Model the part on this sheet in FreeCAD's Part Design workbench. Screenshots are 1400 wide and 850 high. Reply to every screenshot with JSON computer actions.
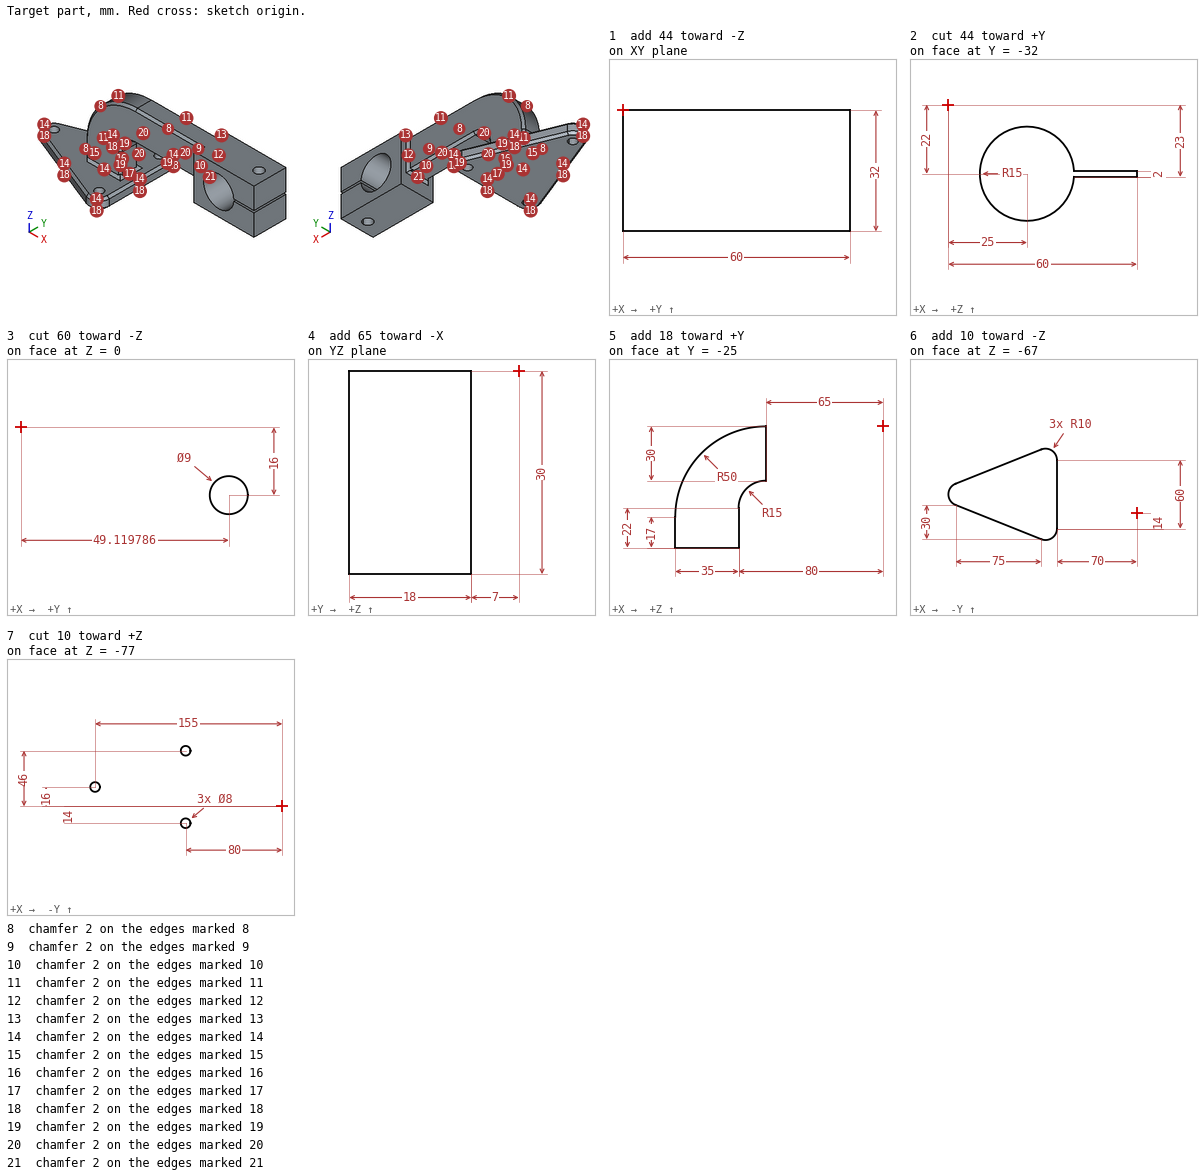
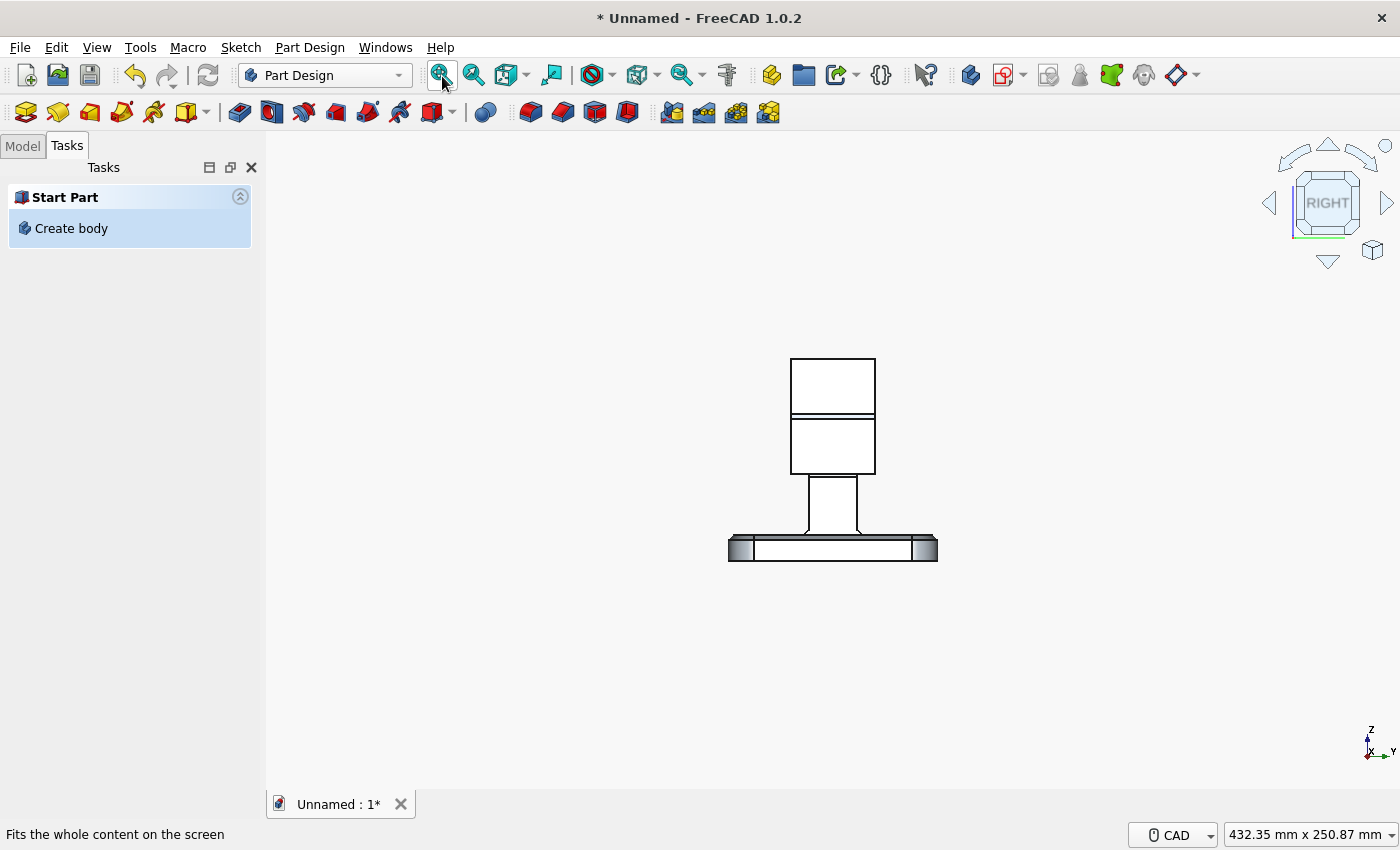
{"action": "key", "text": "5"}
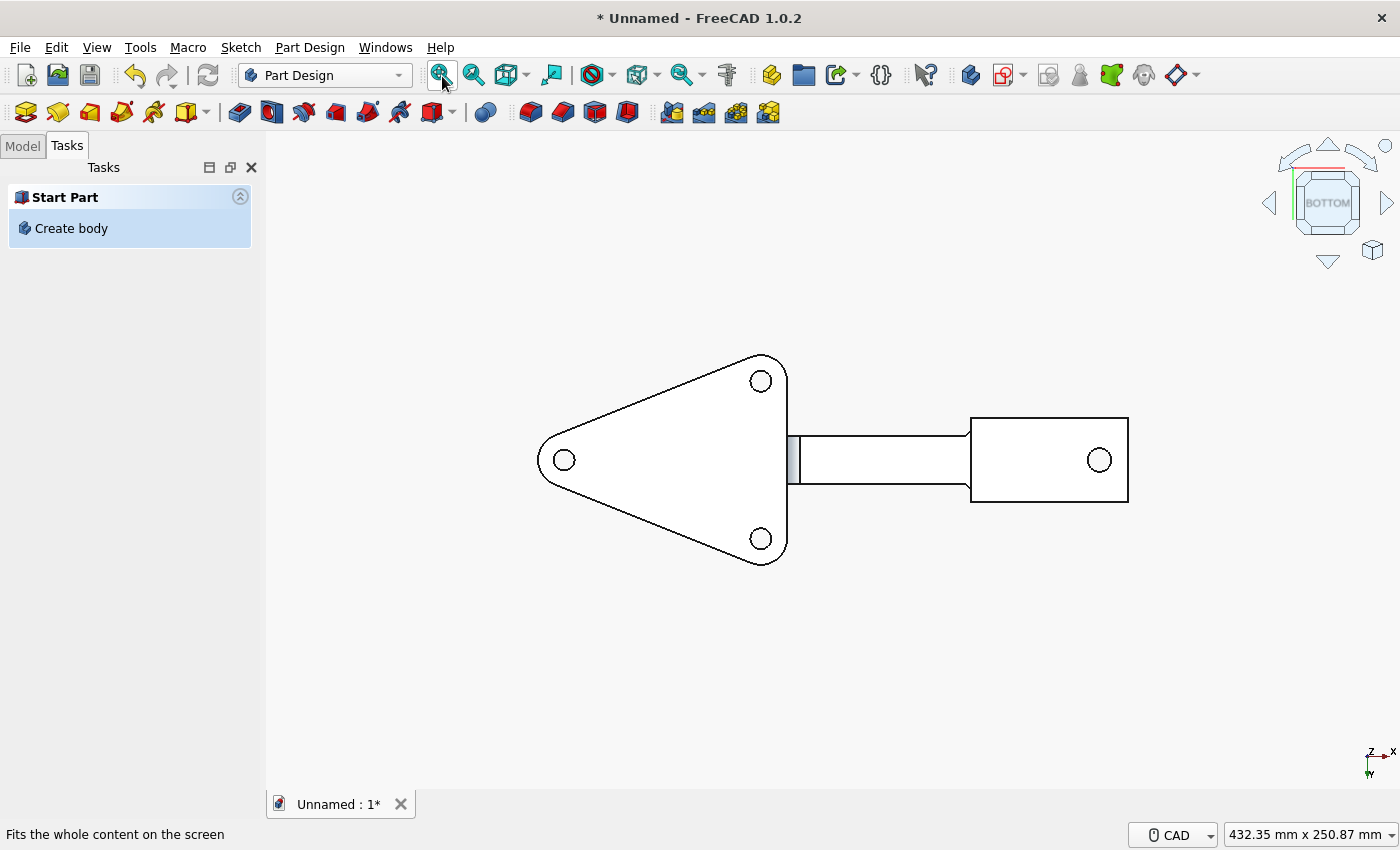
{"action": "key", "text": "4"}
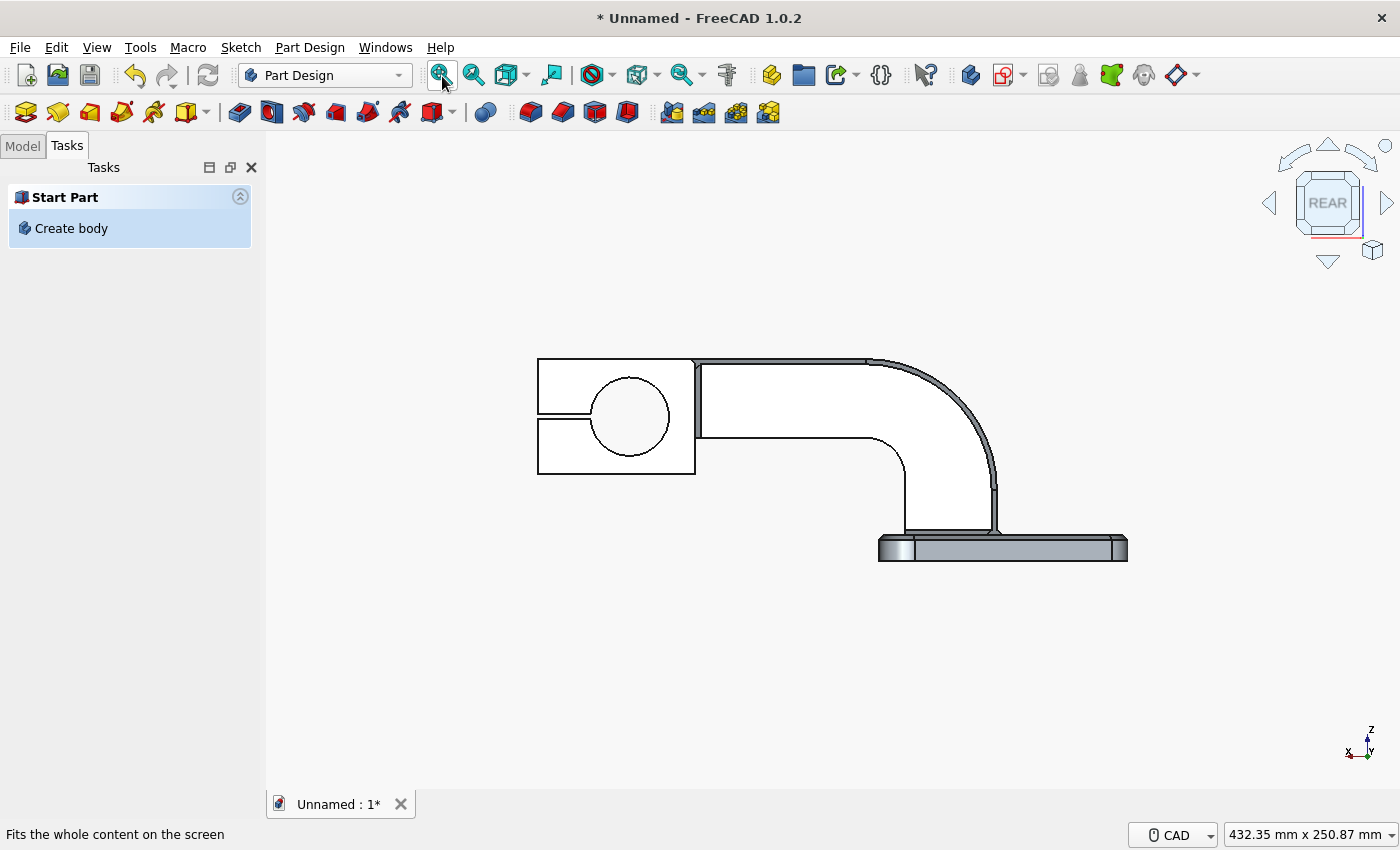
{"action": "key", "text": "6"}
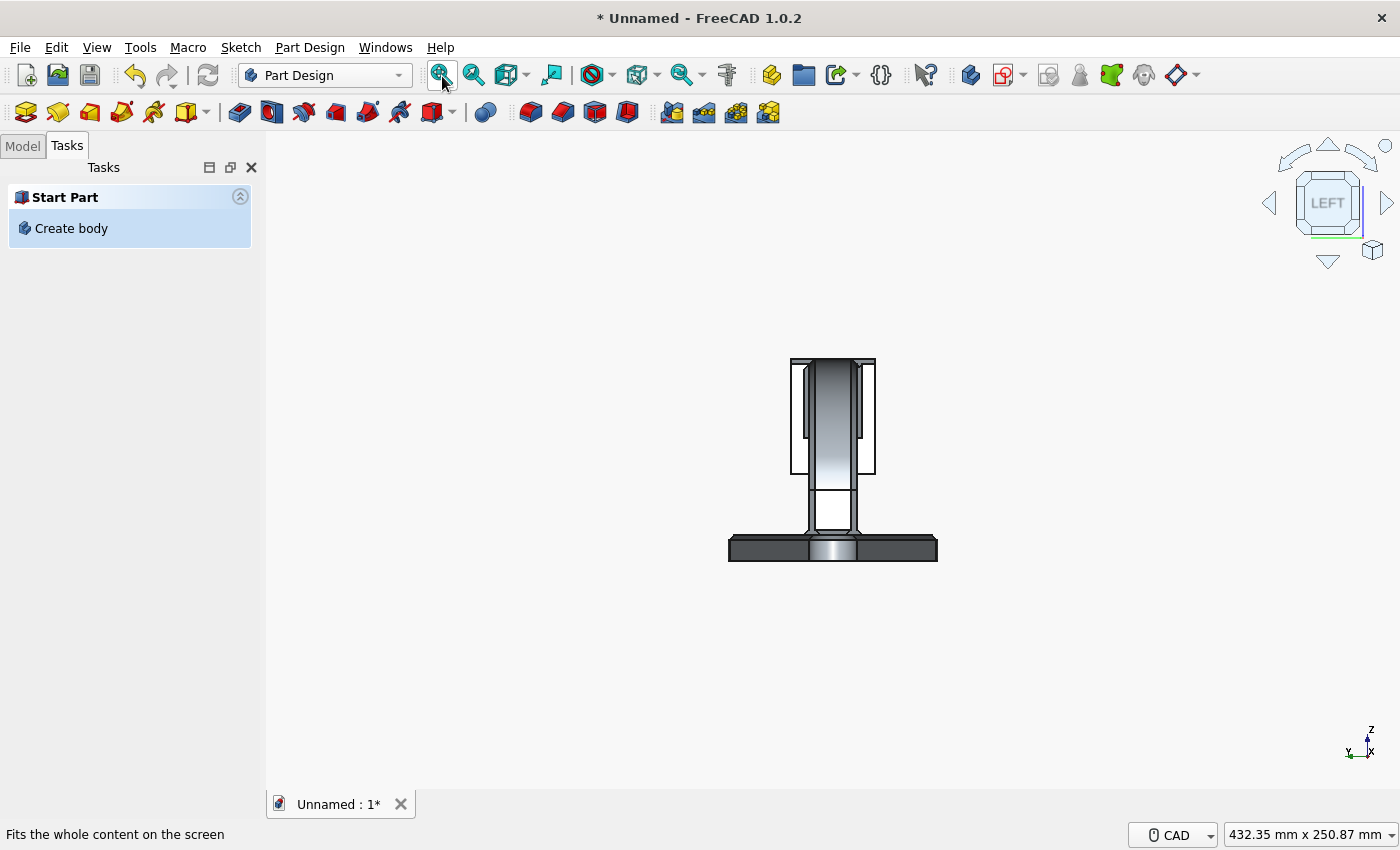
{"action": "left_click", "coordinate": [442, 76]}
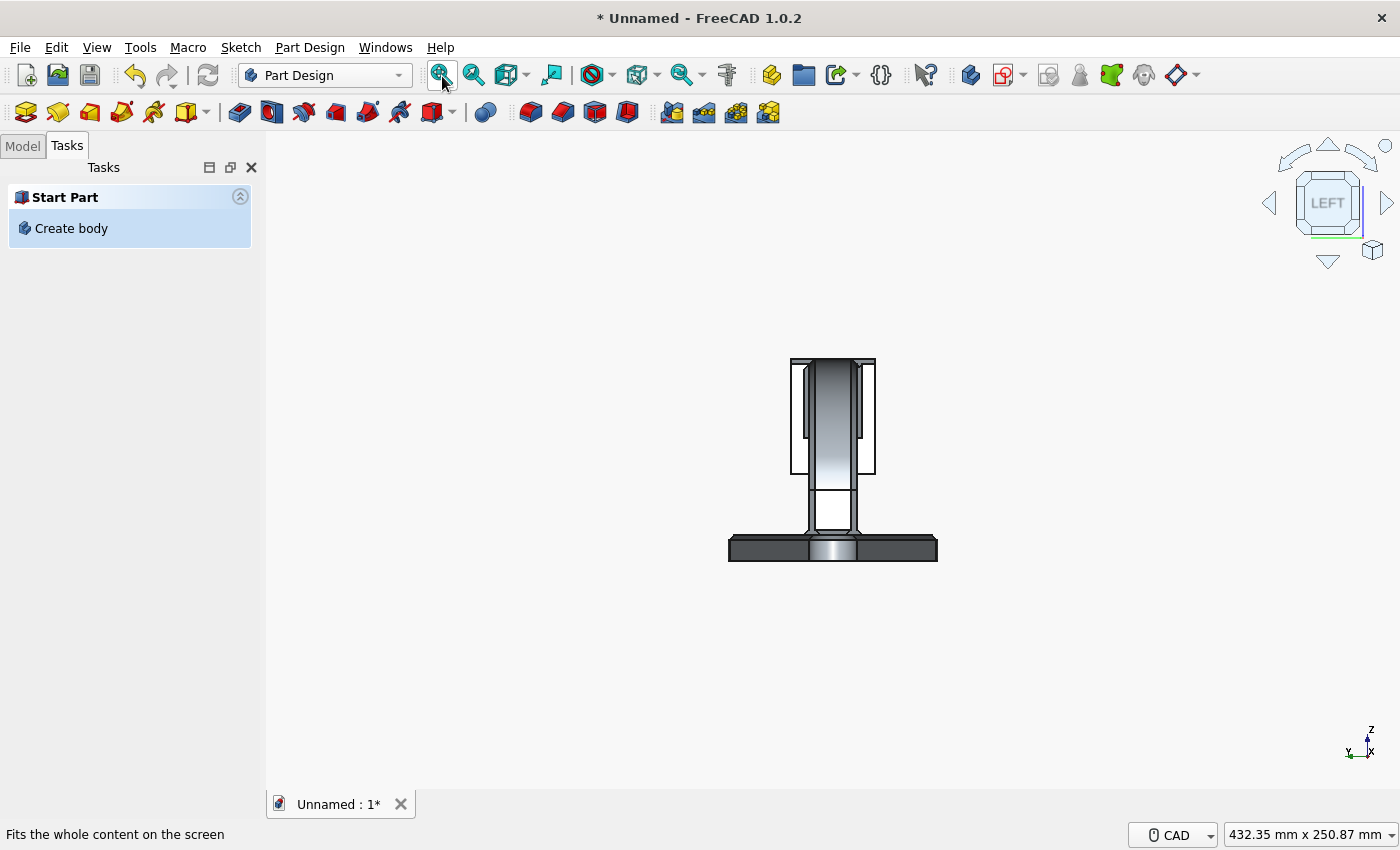
{"action": "key", "text": "v 3"}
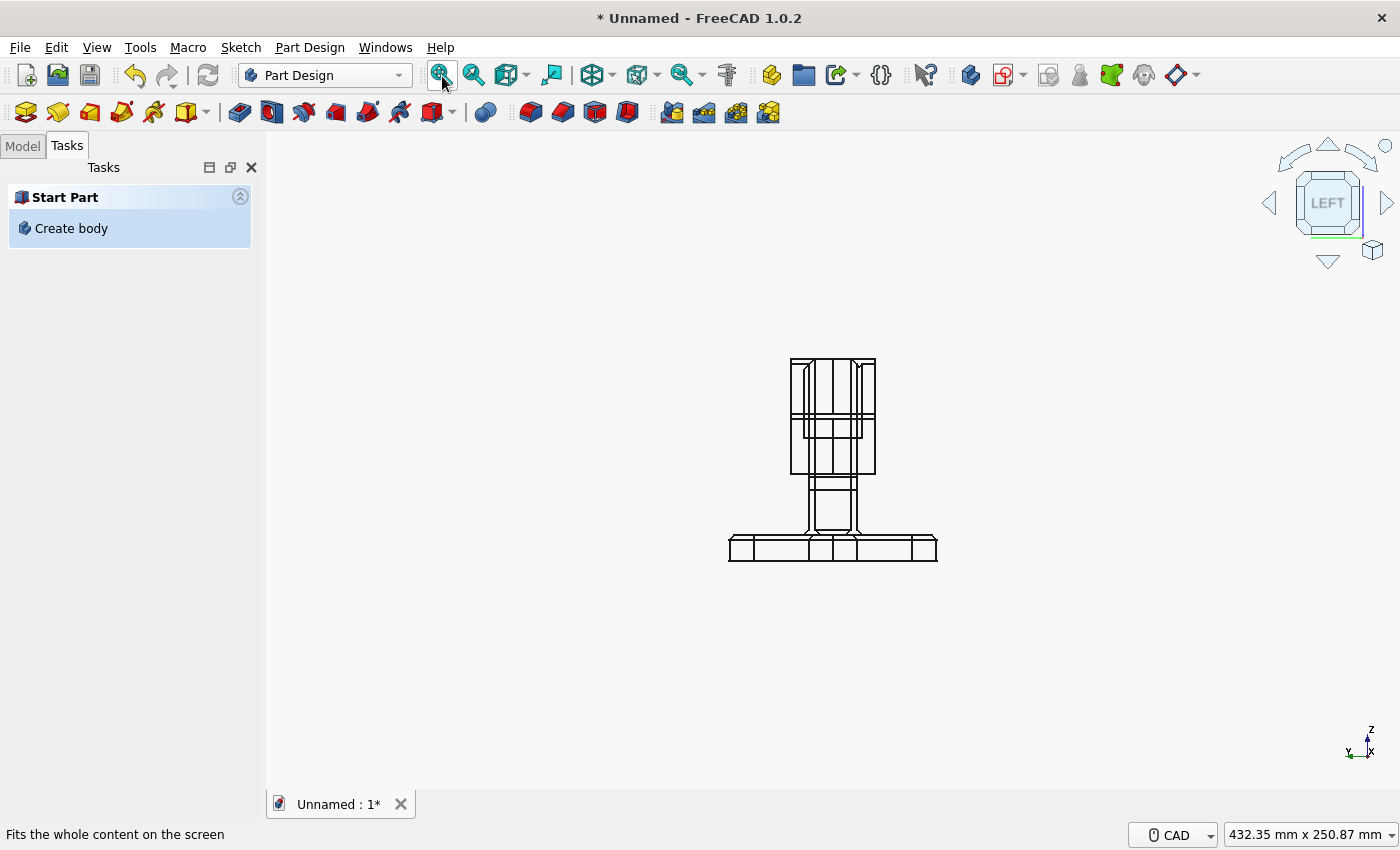
{"action": "key", "text": "0"}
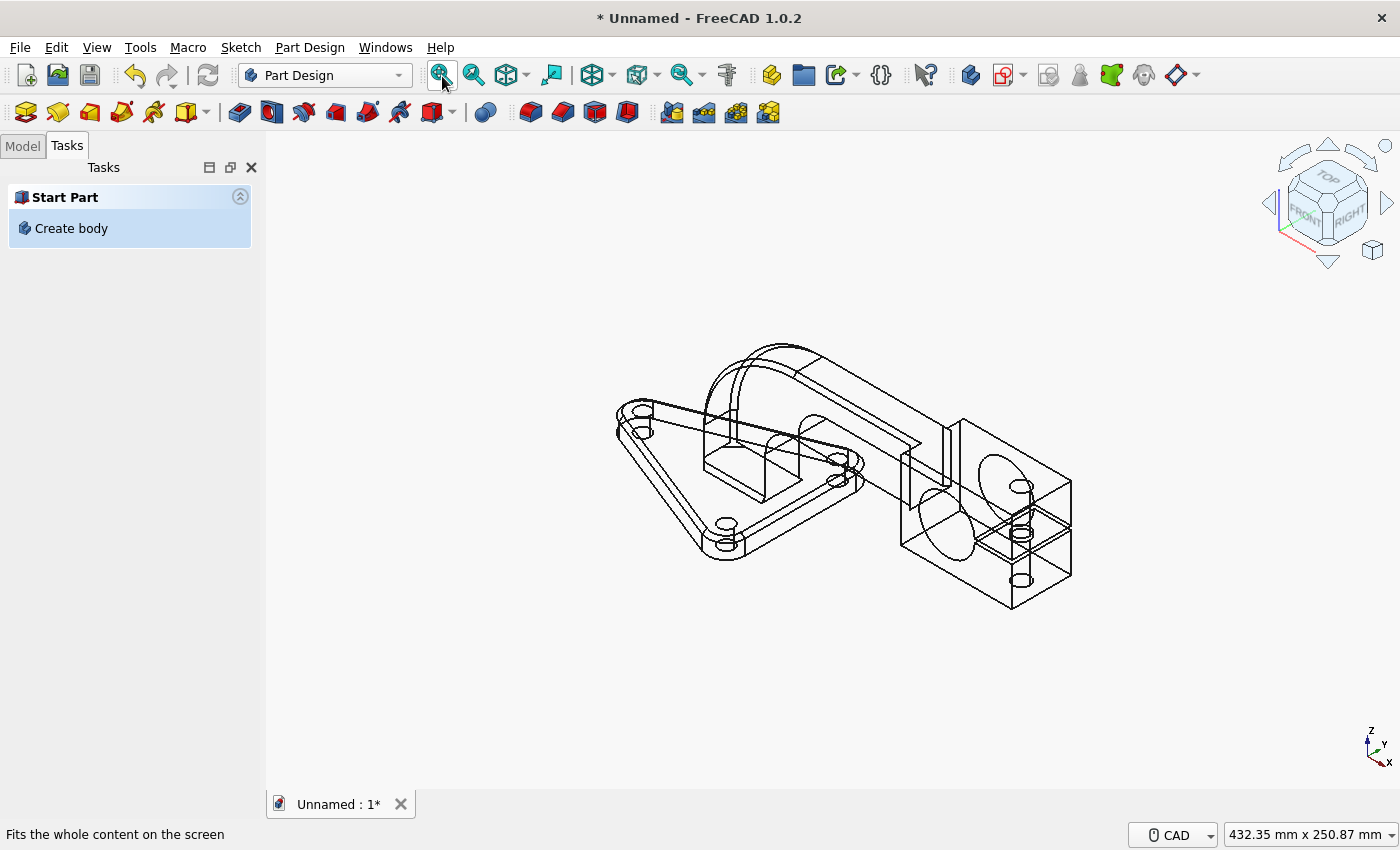
{"action": "left_click", "coordinate": [782, 491]}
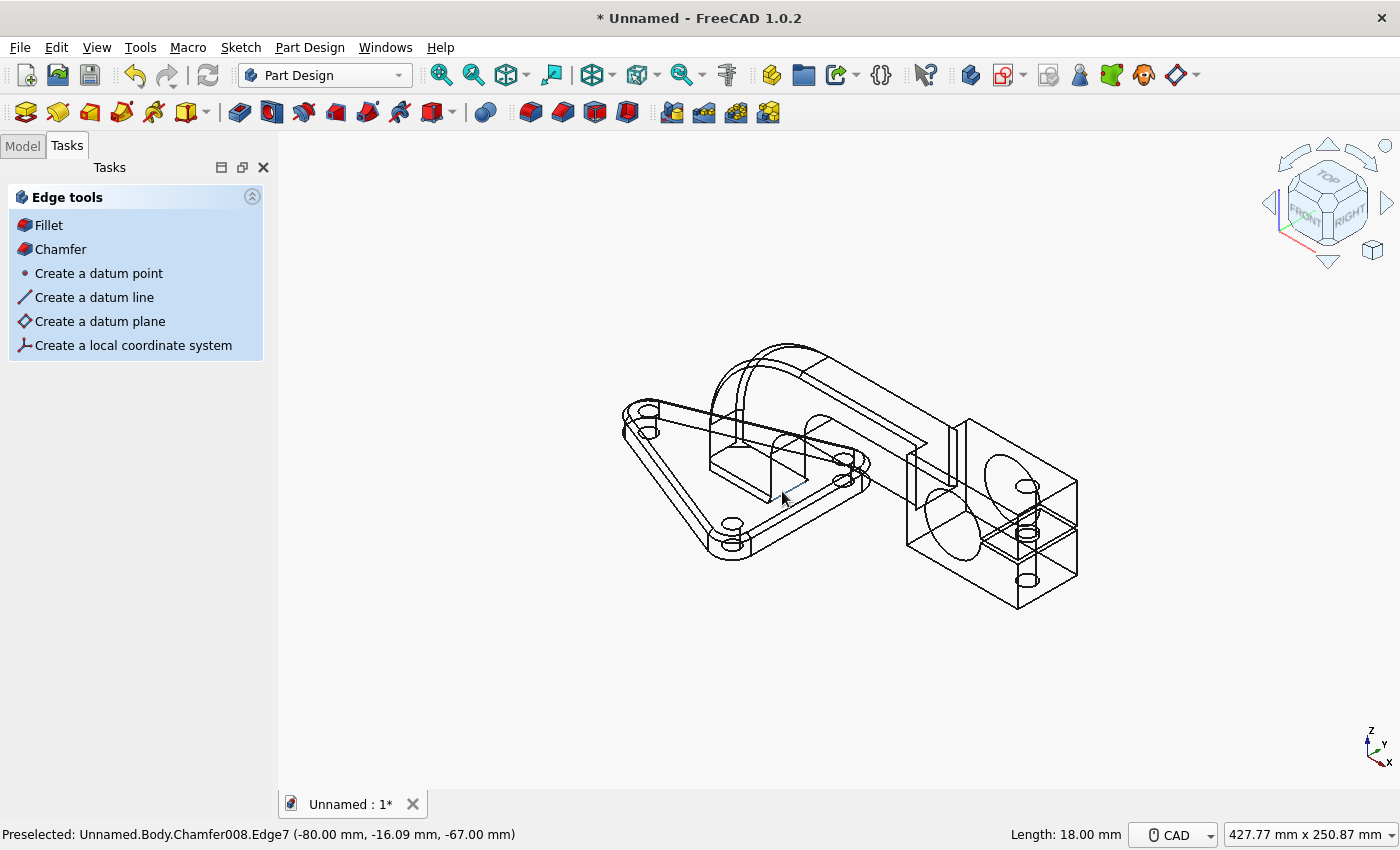
{"action": "key", "text": "v 1"}